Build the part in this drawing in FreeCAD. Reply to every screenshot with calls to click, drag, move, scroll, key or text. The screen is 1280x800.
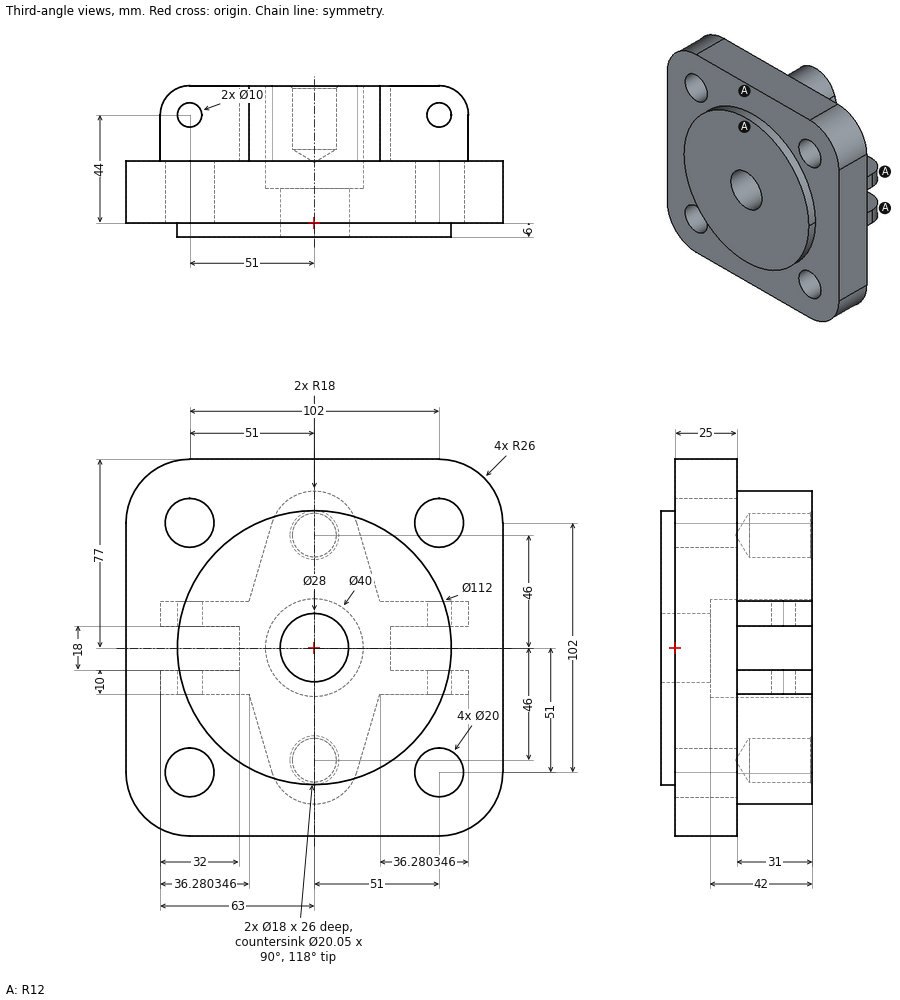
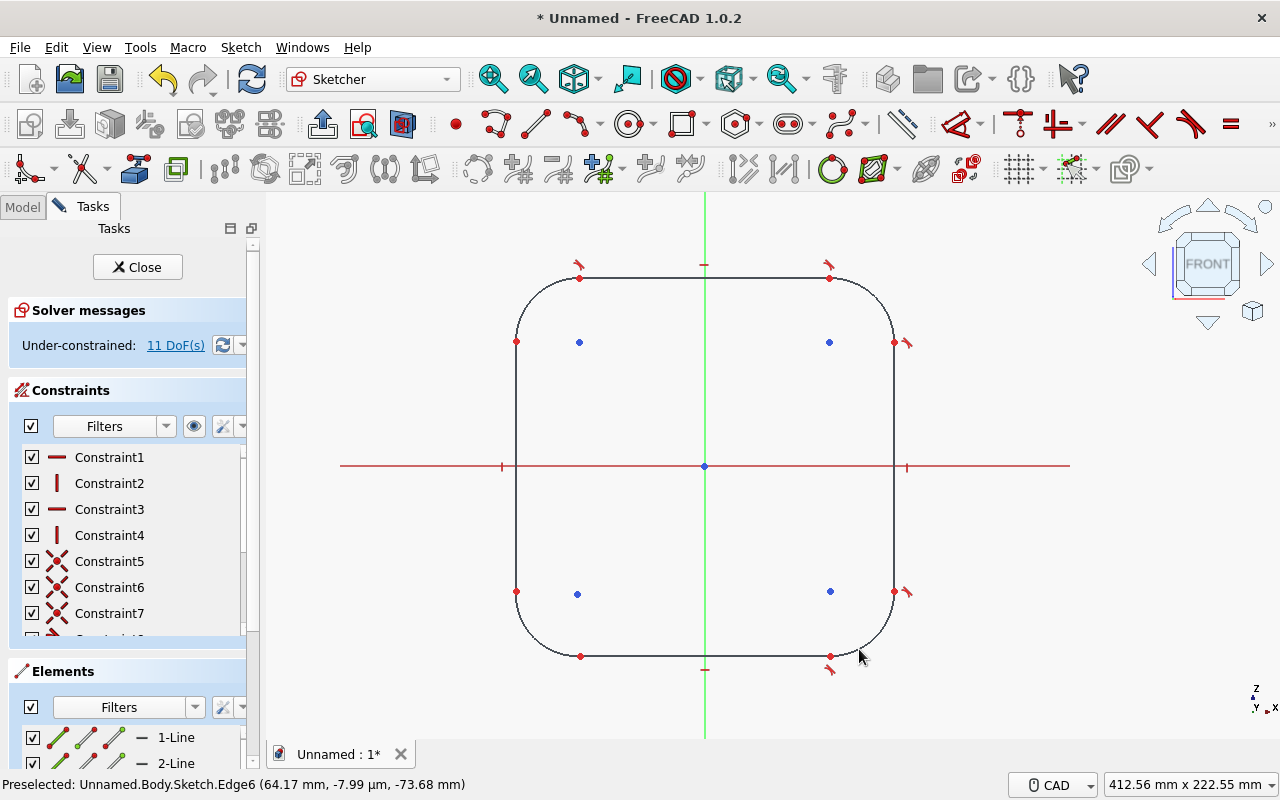
click(755, 656)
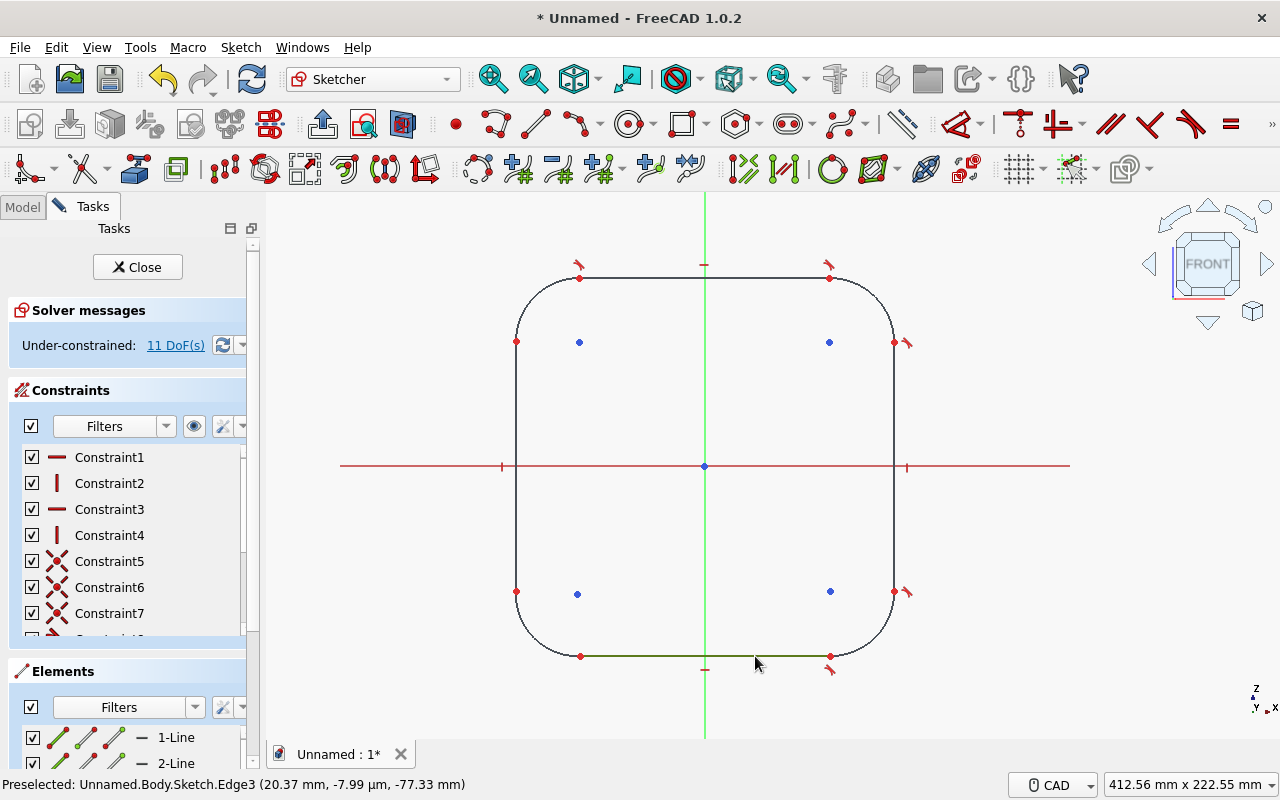
click(522, 622)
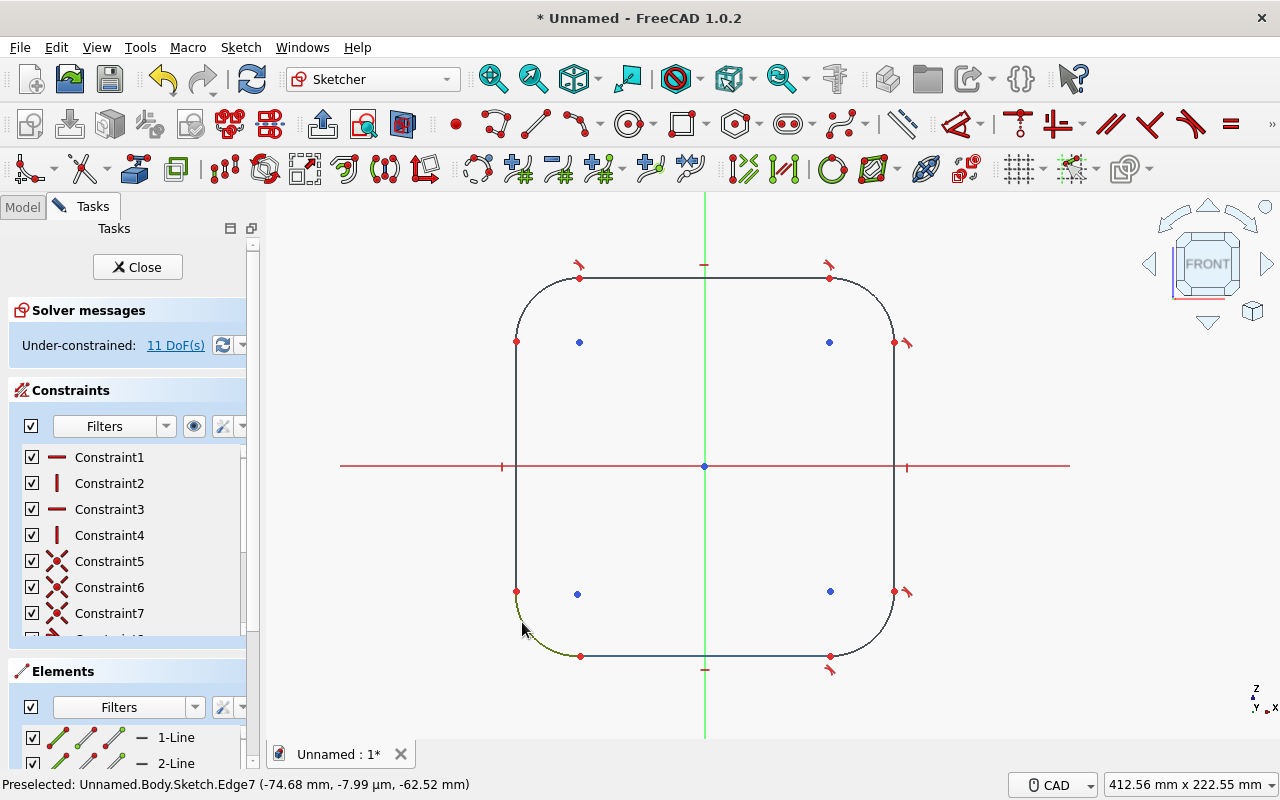
key(t)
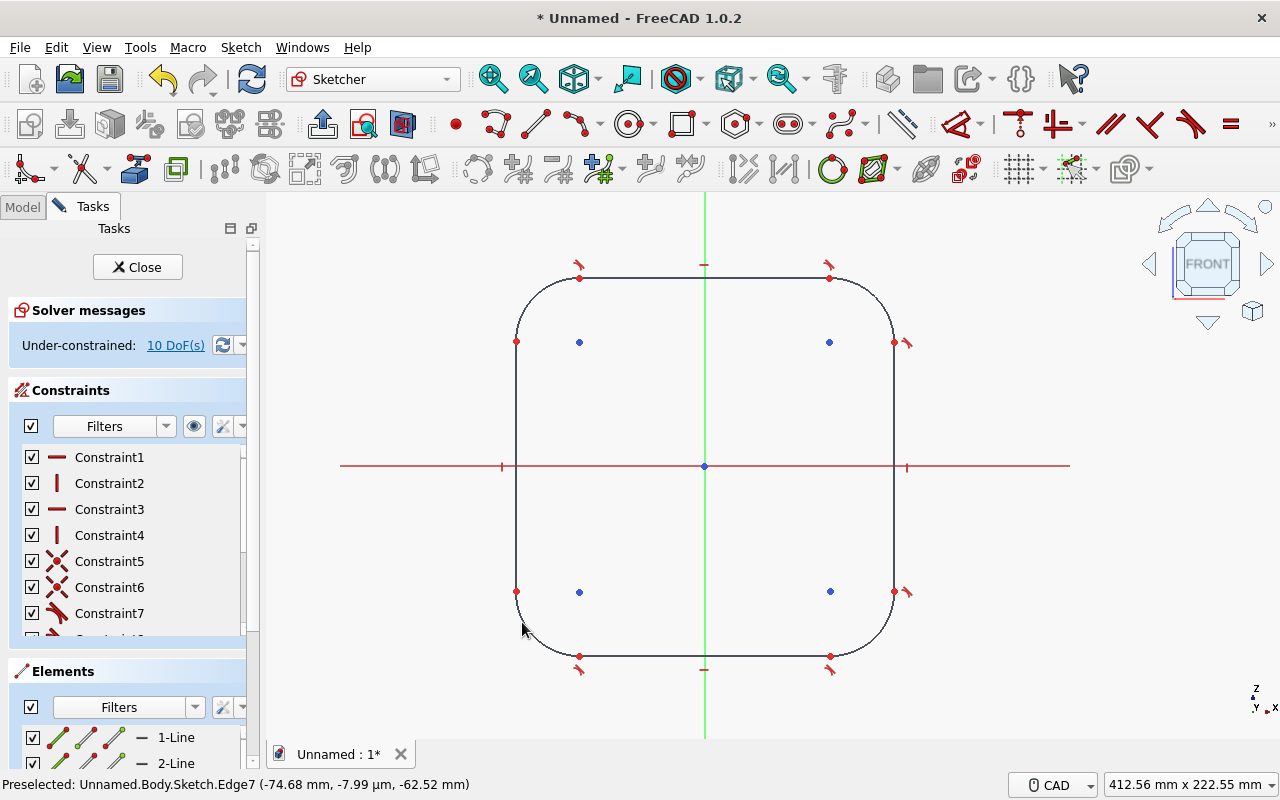
click(516, 517)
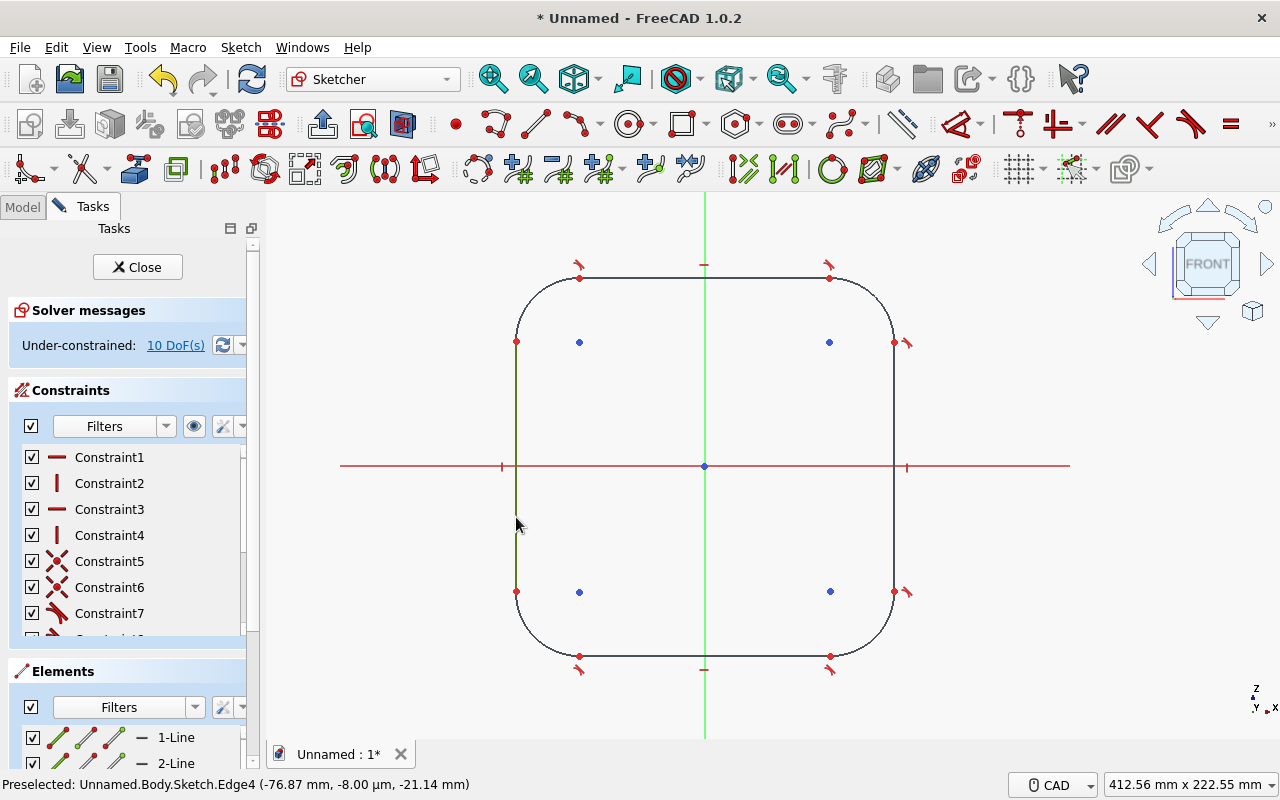
click(523, 621)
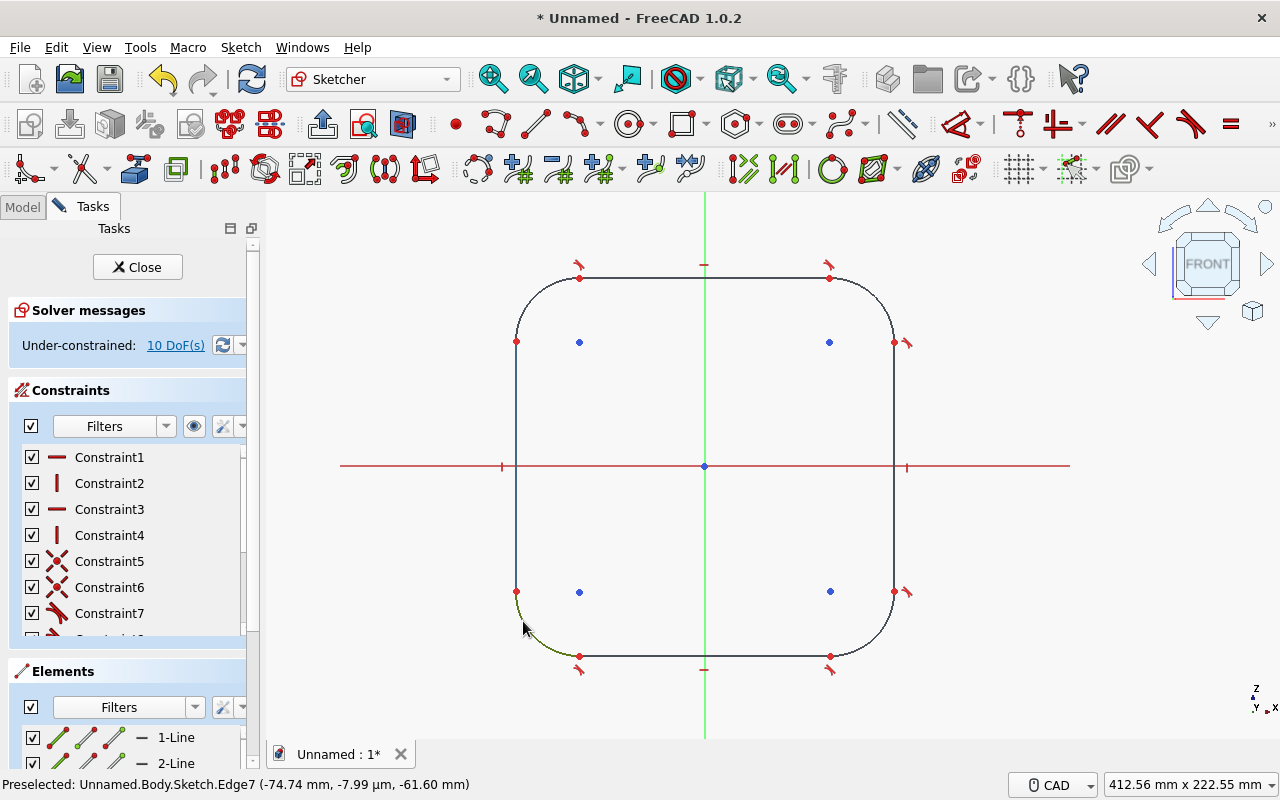
key(t)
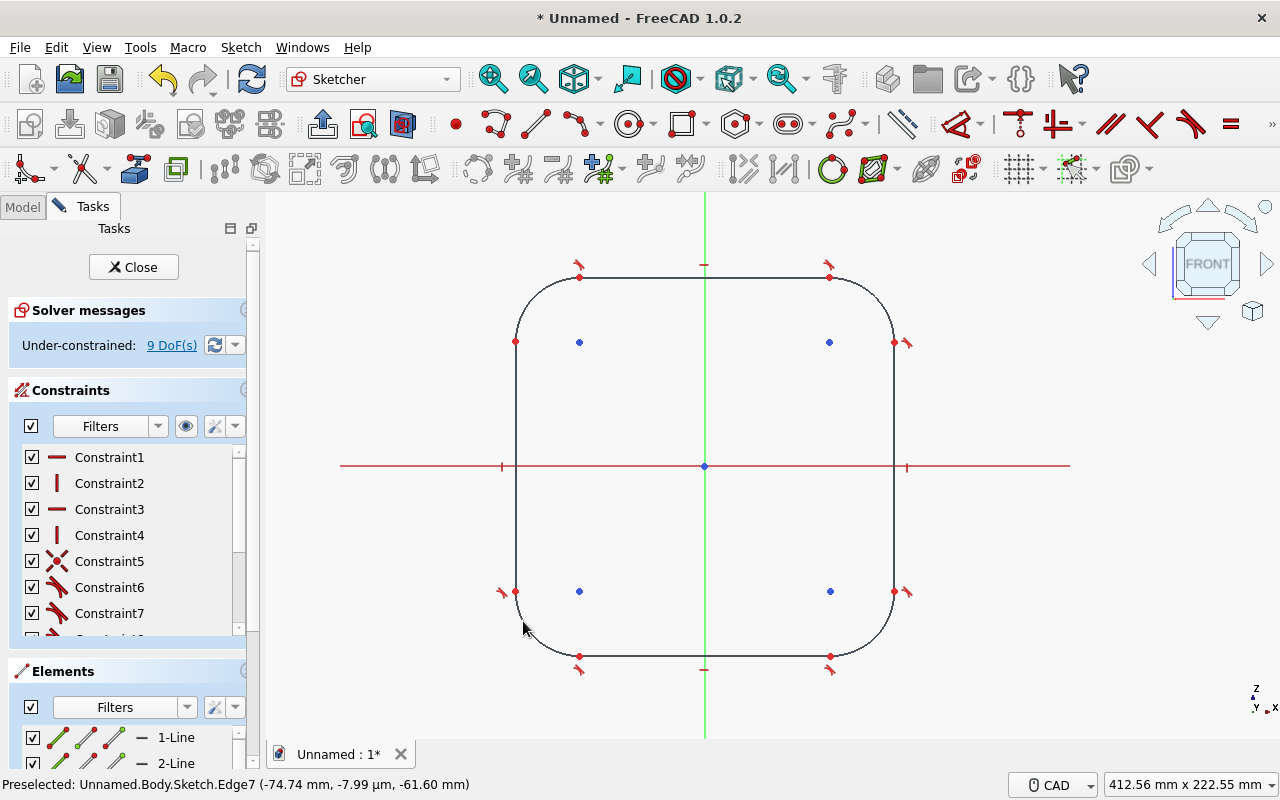
click(516, 517)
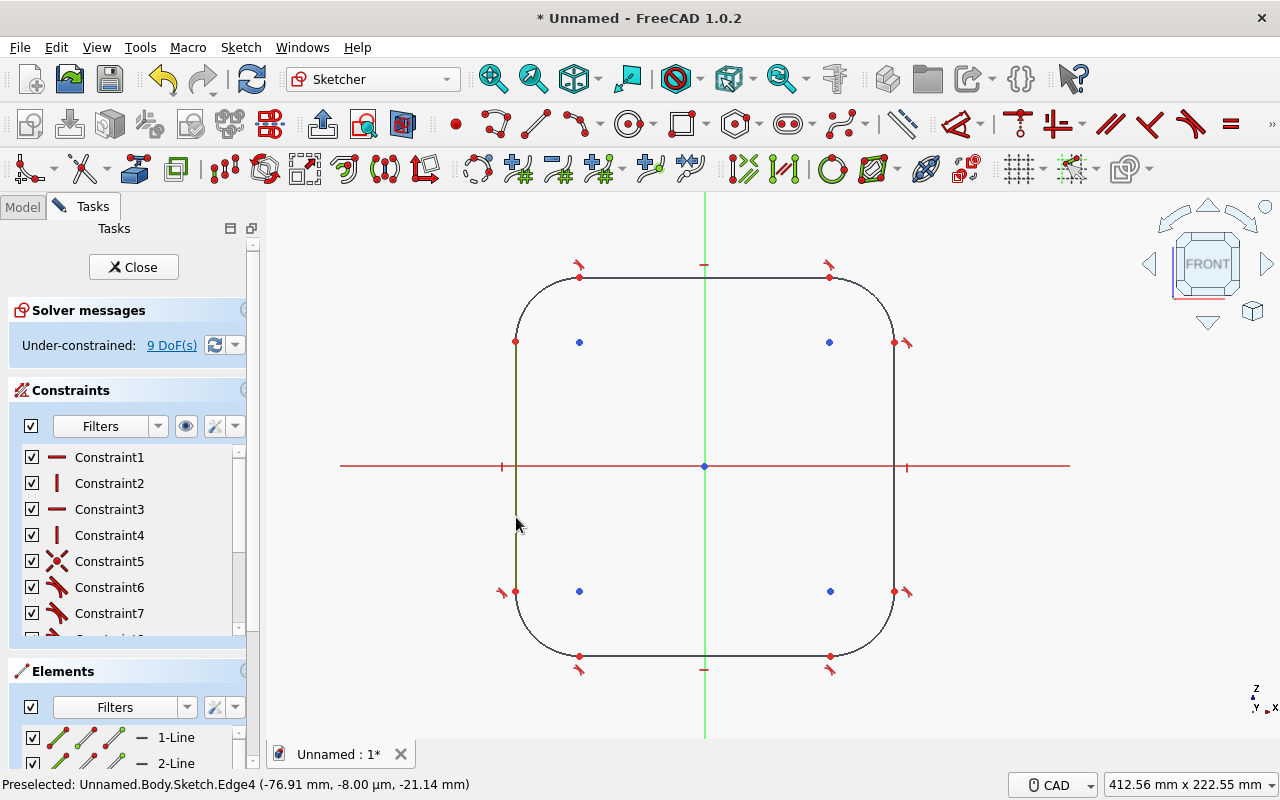
click(551, 285)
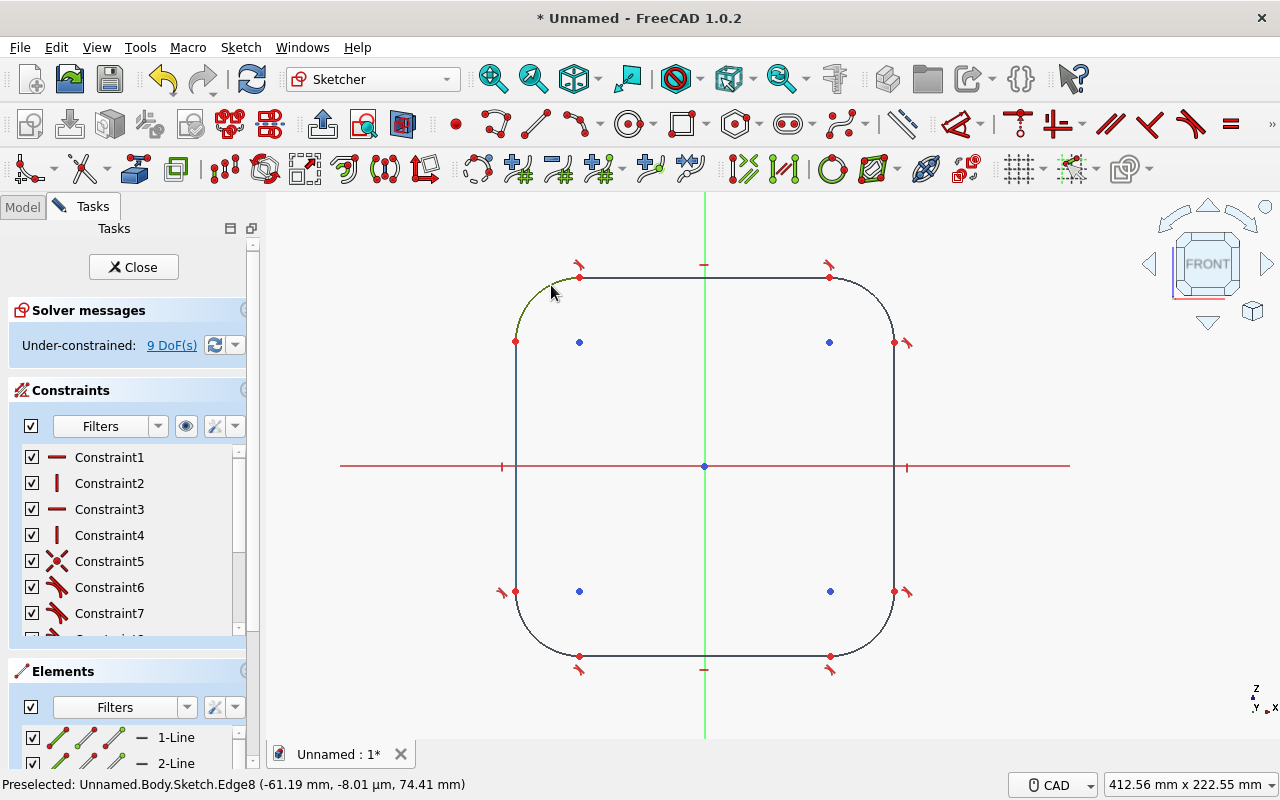
key(t)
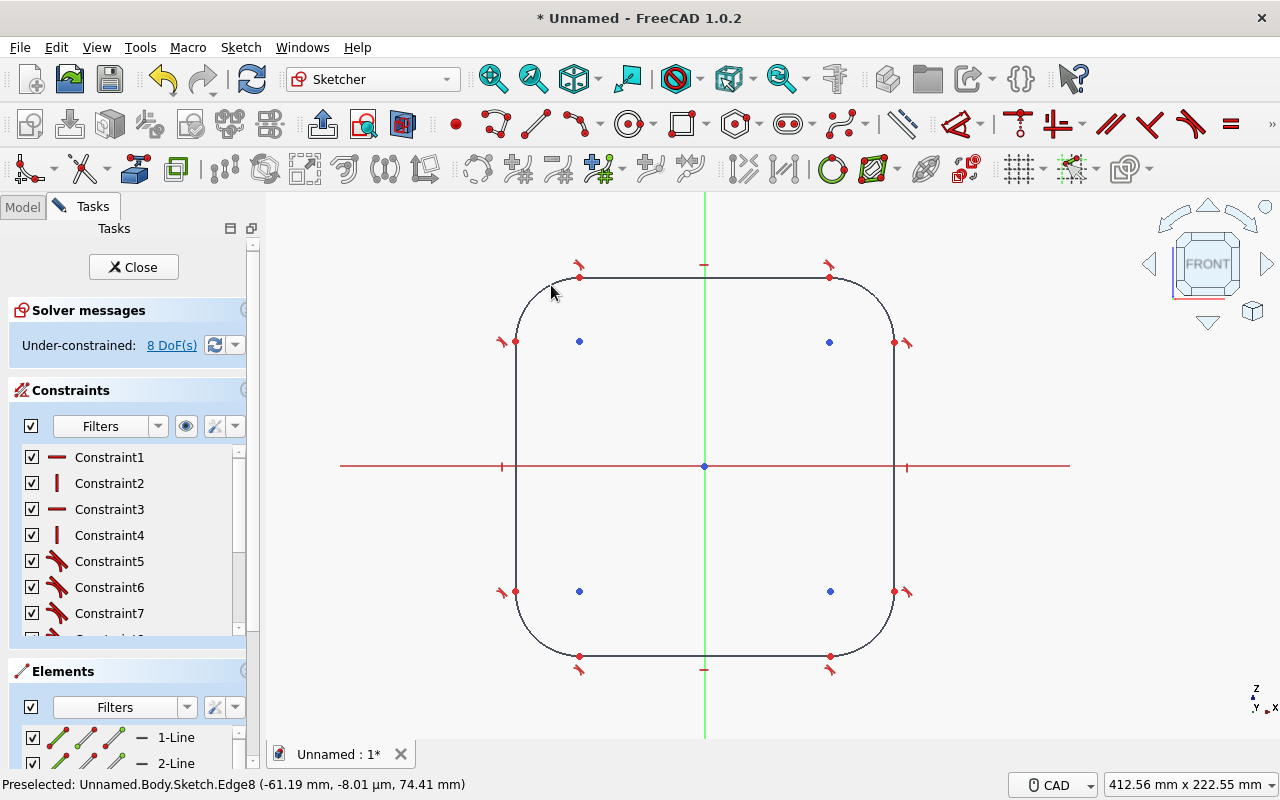
click(887, 313)